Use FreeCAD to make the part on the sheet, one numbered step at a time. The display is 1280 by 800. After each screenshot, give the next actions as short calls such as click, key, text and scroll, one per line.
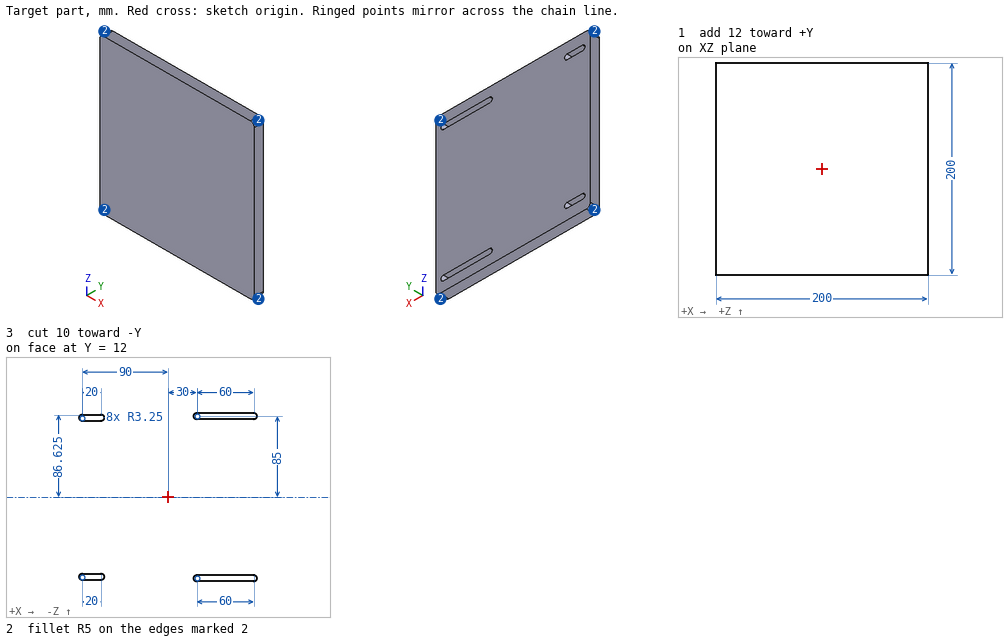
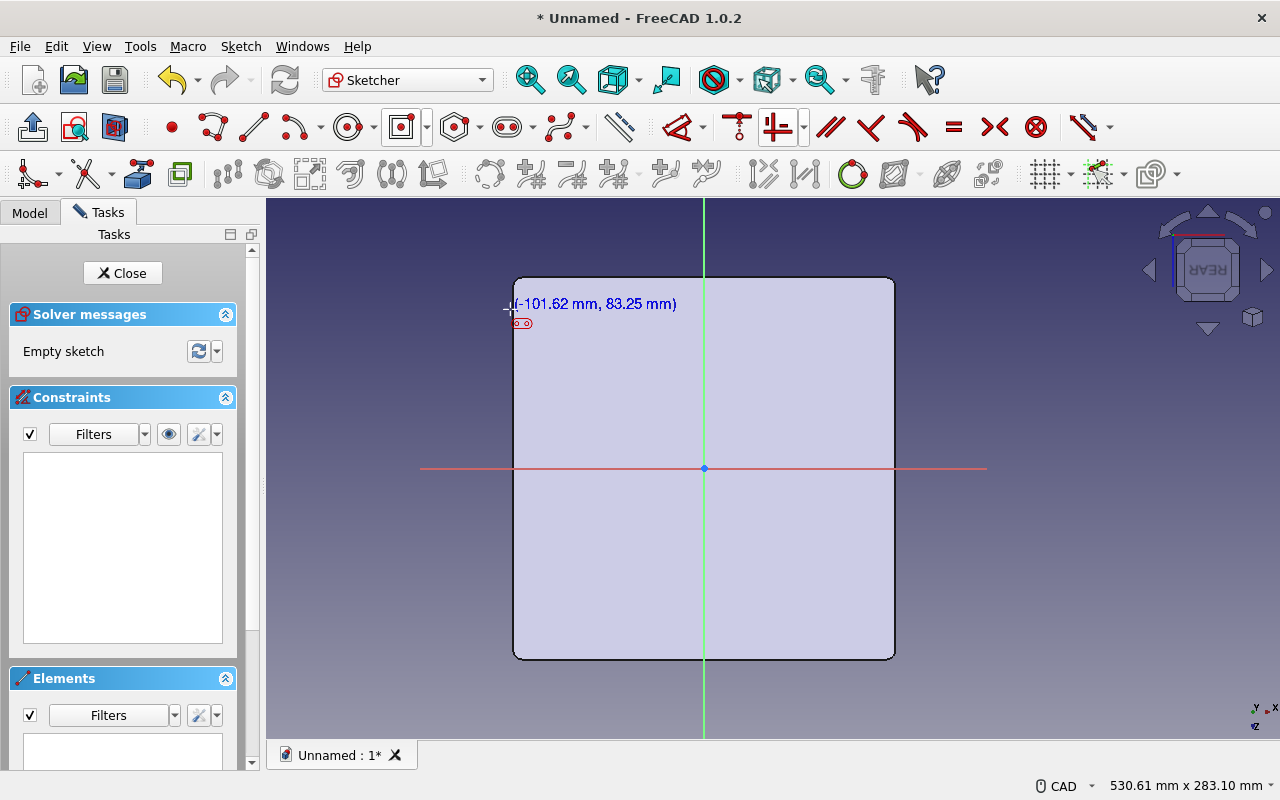
click(532, 309)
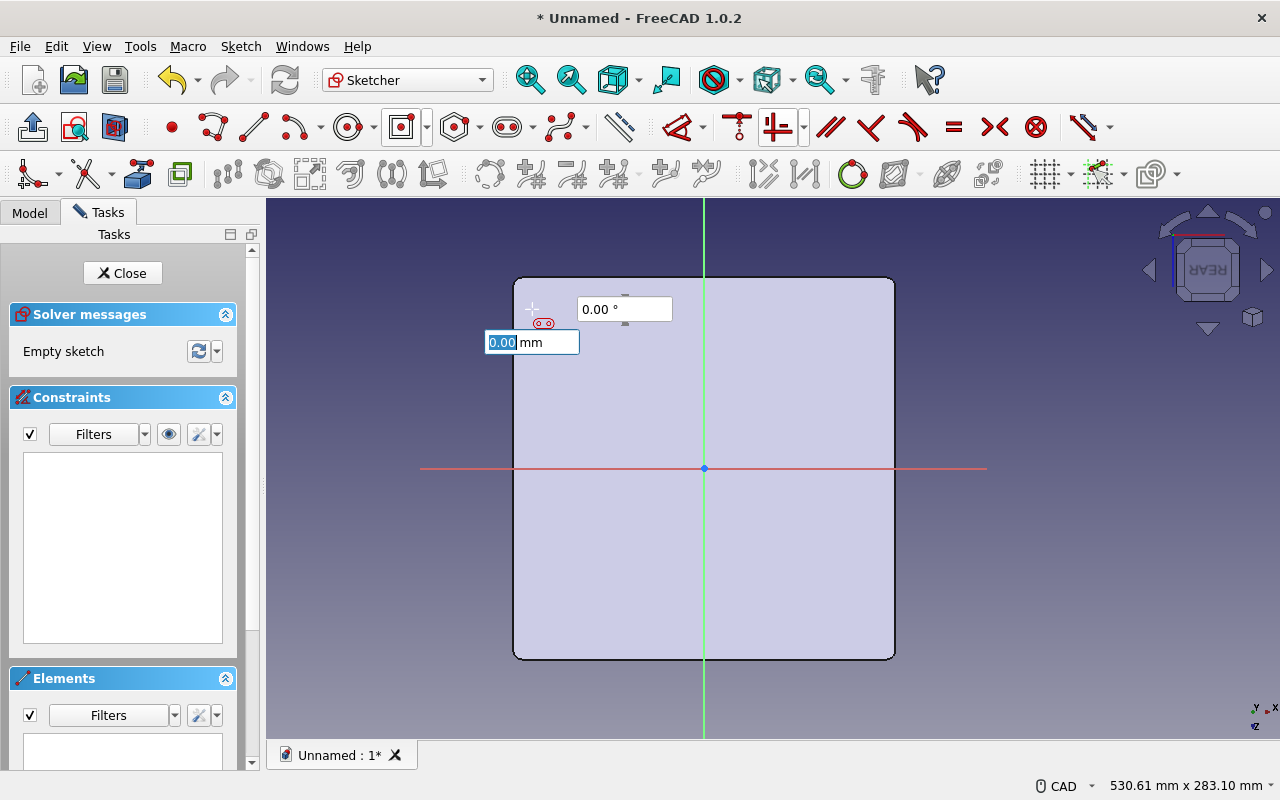
click(571, 309)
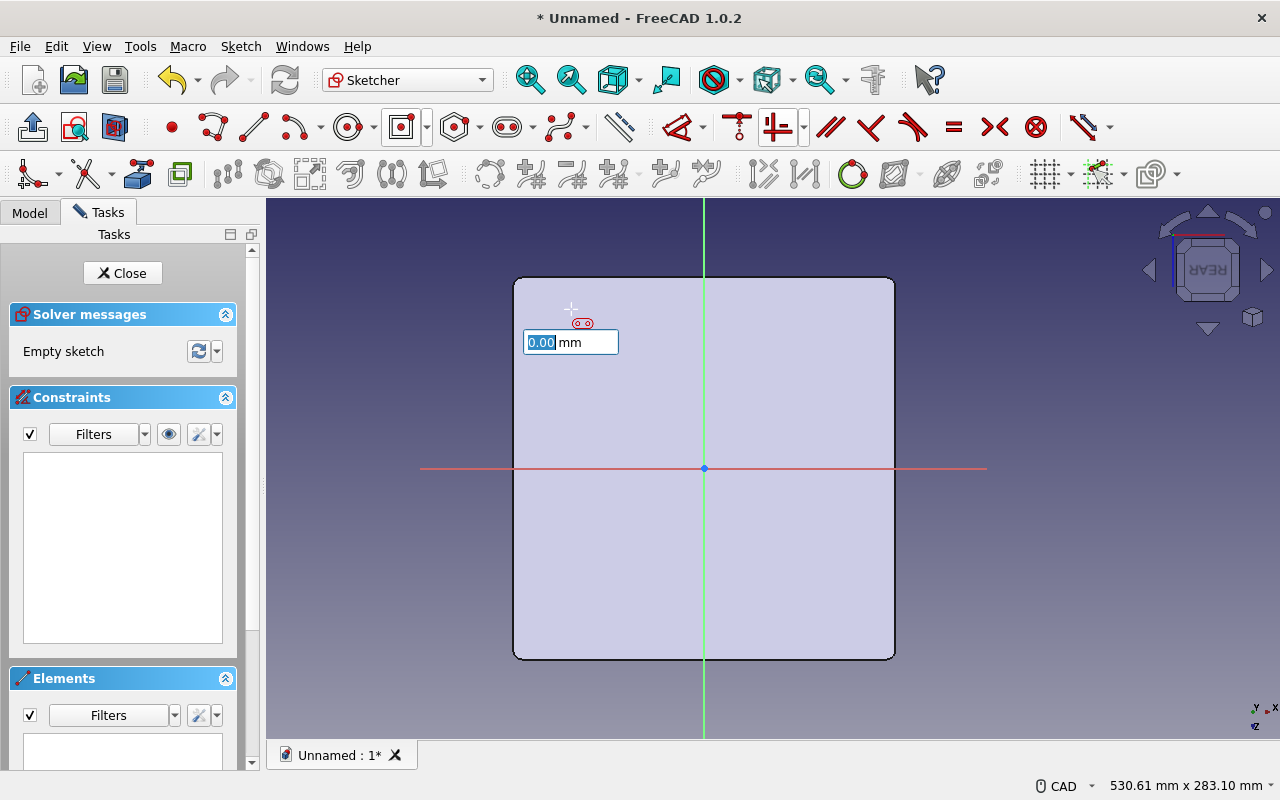
scroll(551, 303, up, 5)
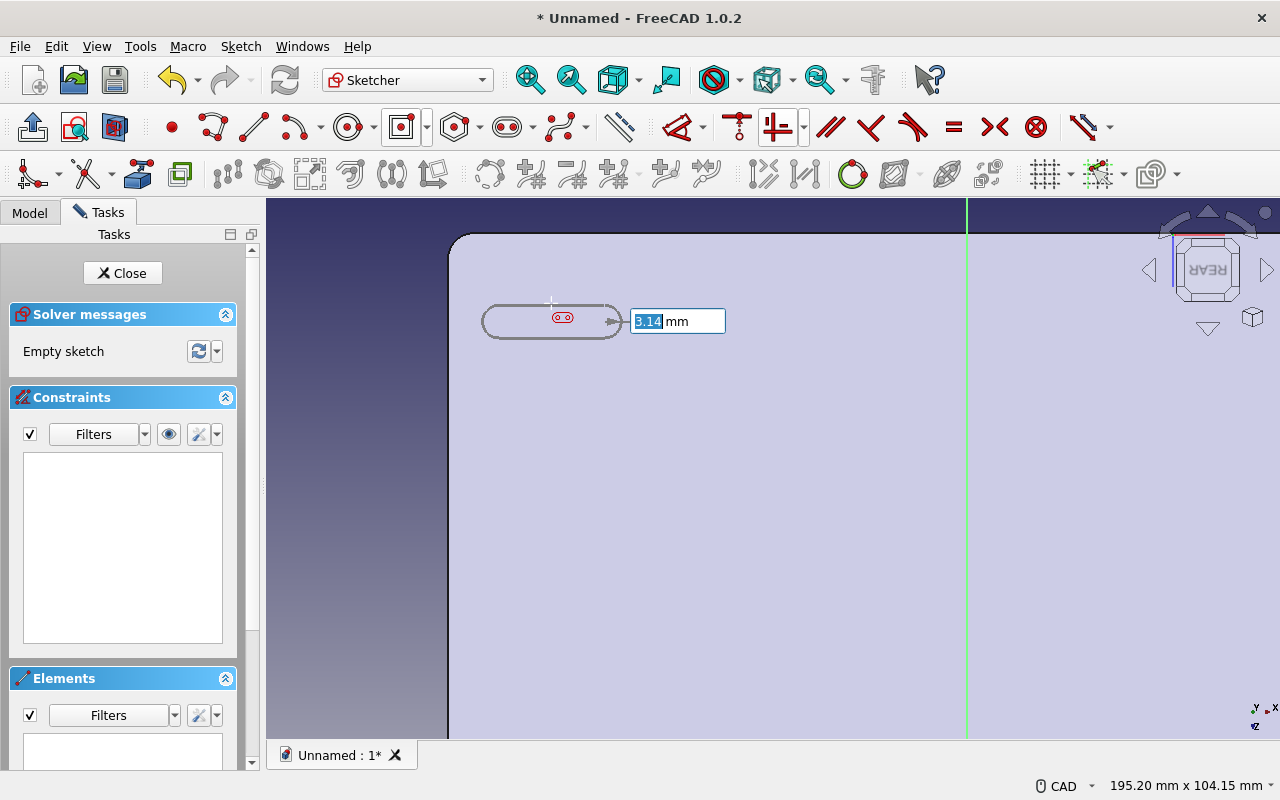
click(552, 303)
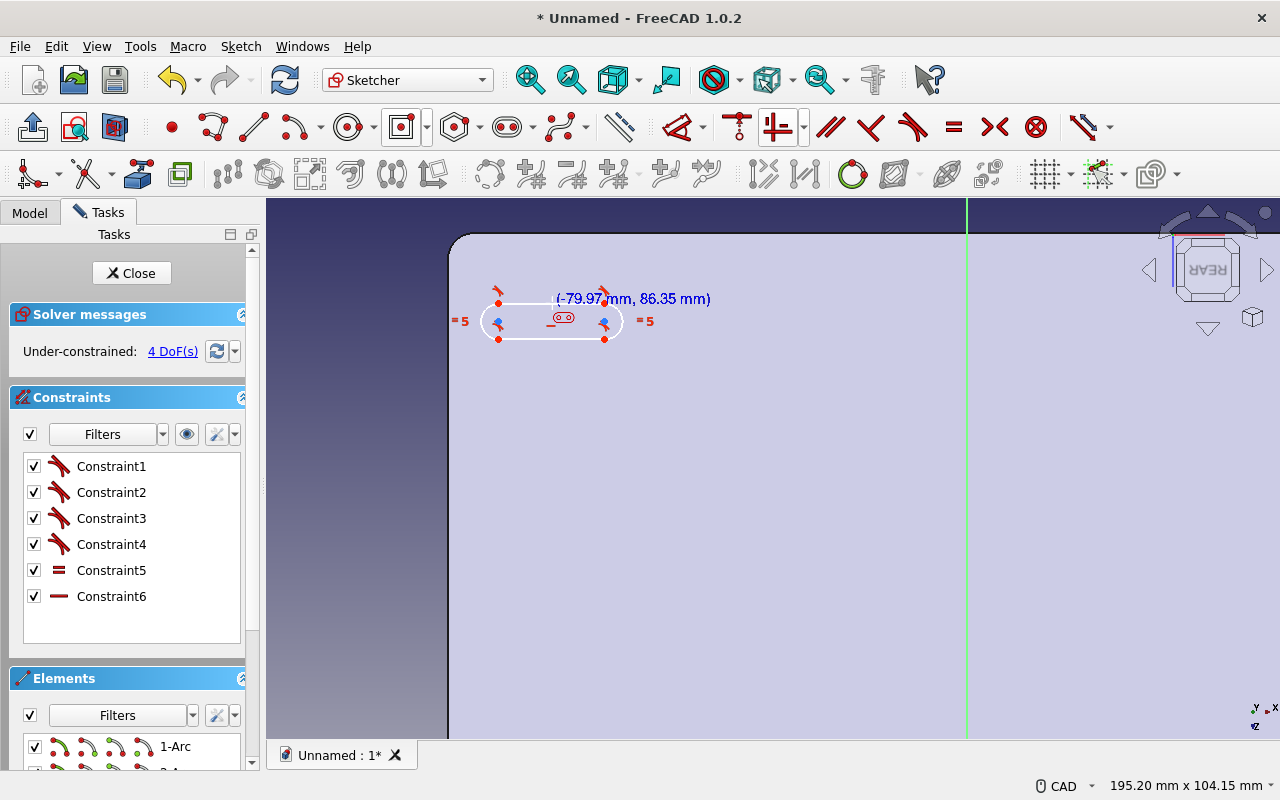
scroll(551, 303, down, 5)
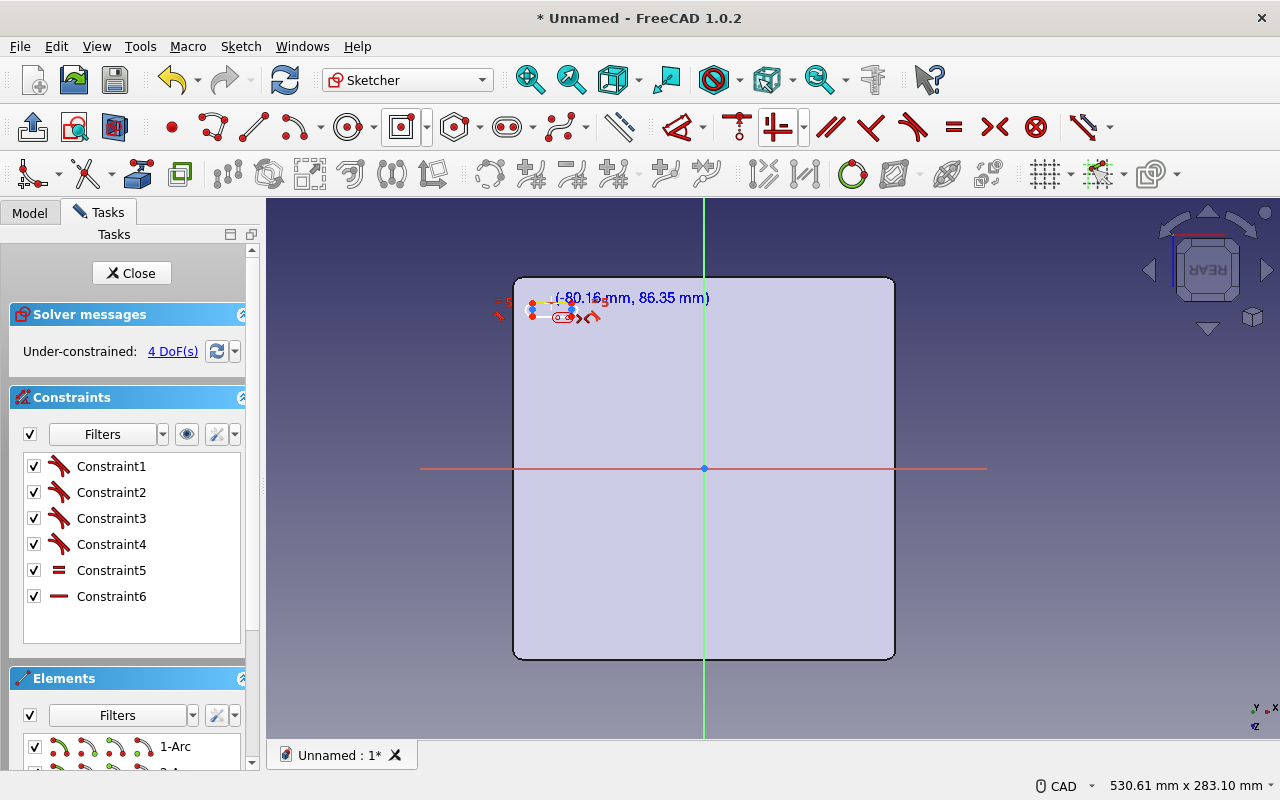
scroll(532, 628, up, 7)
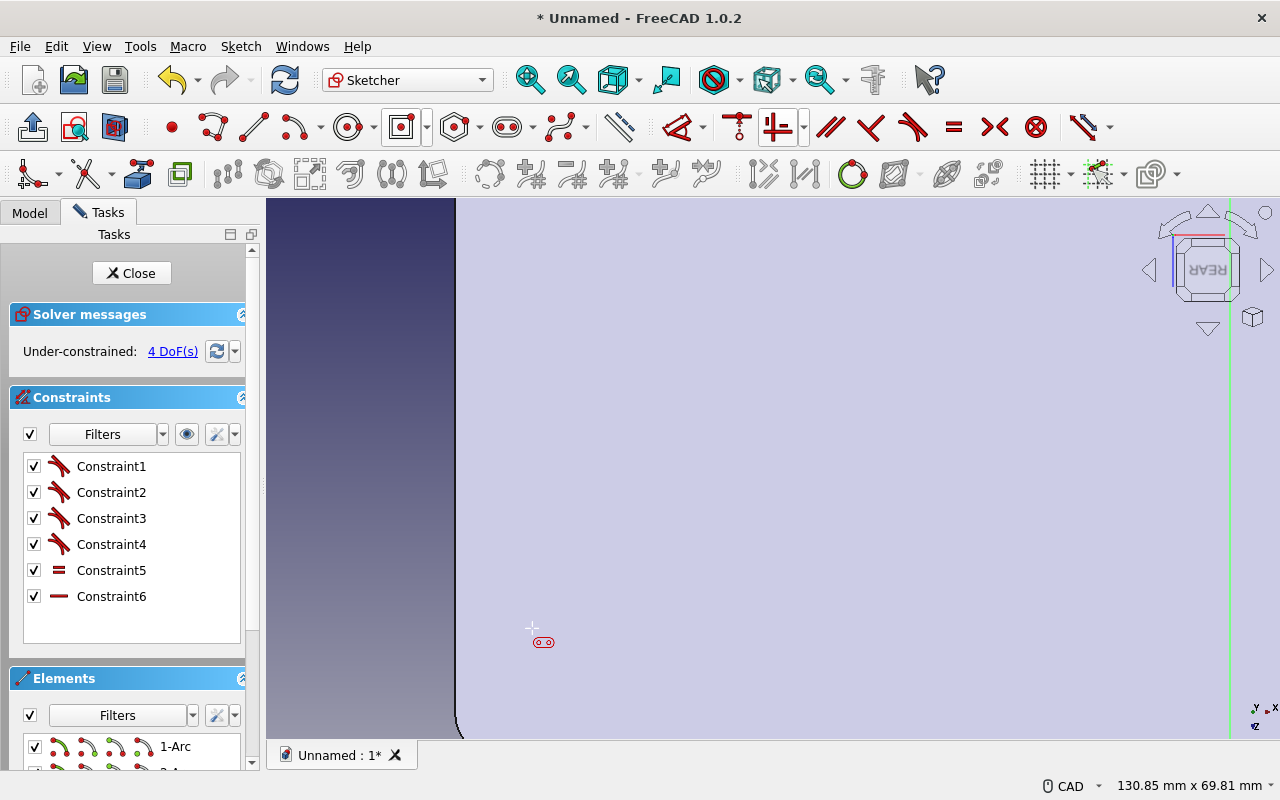
scroll(532, 629, down, 7)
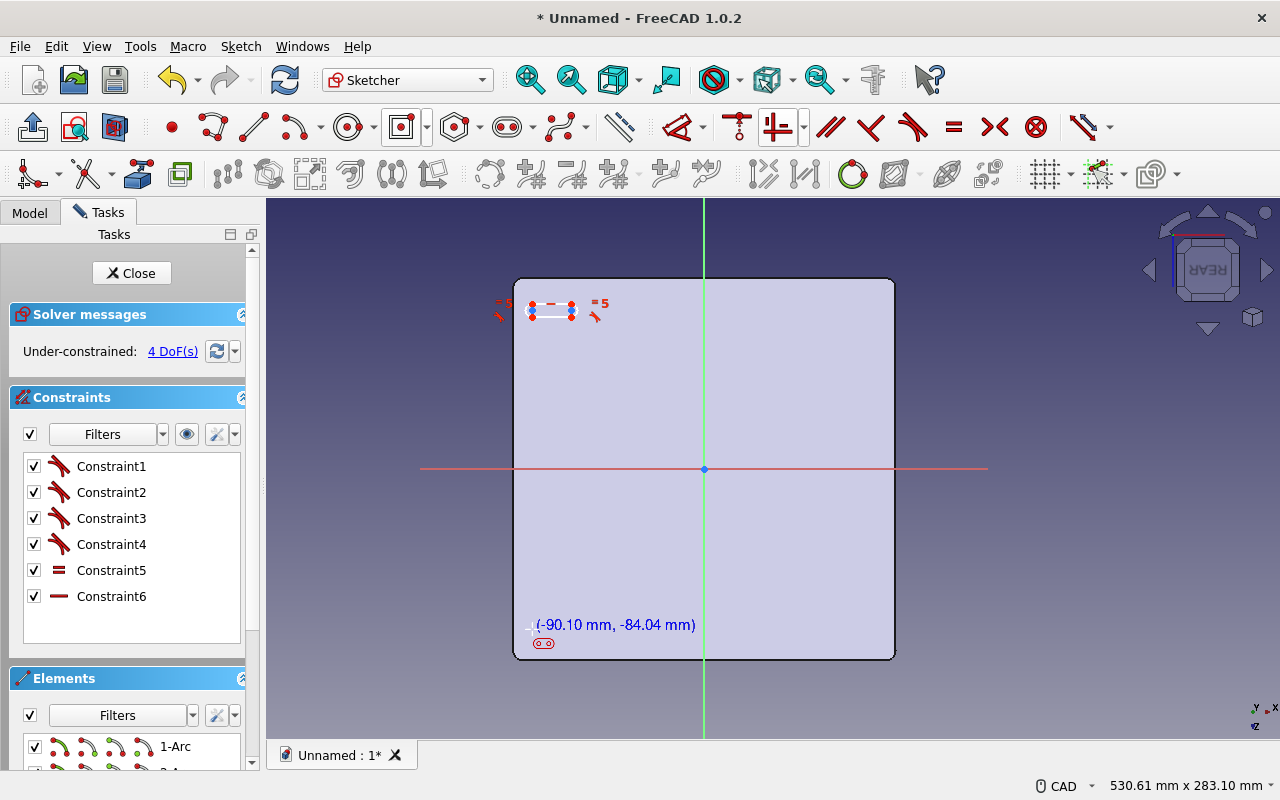
click(532, 629)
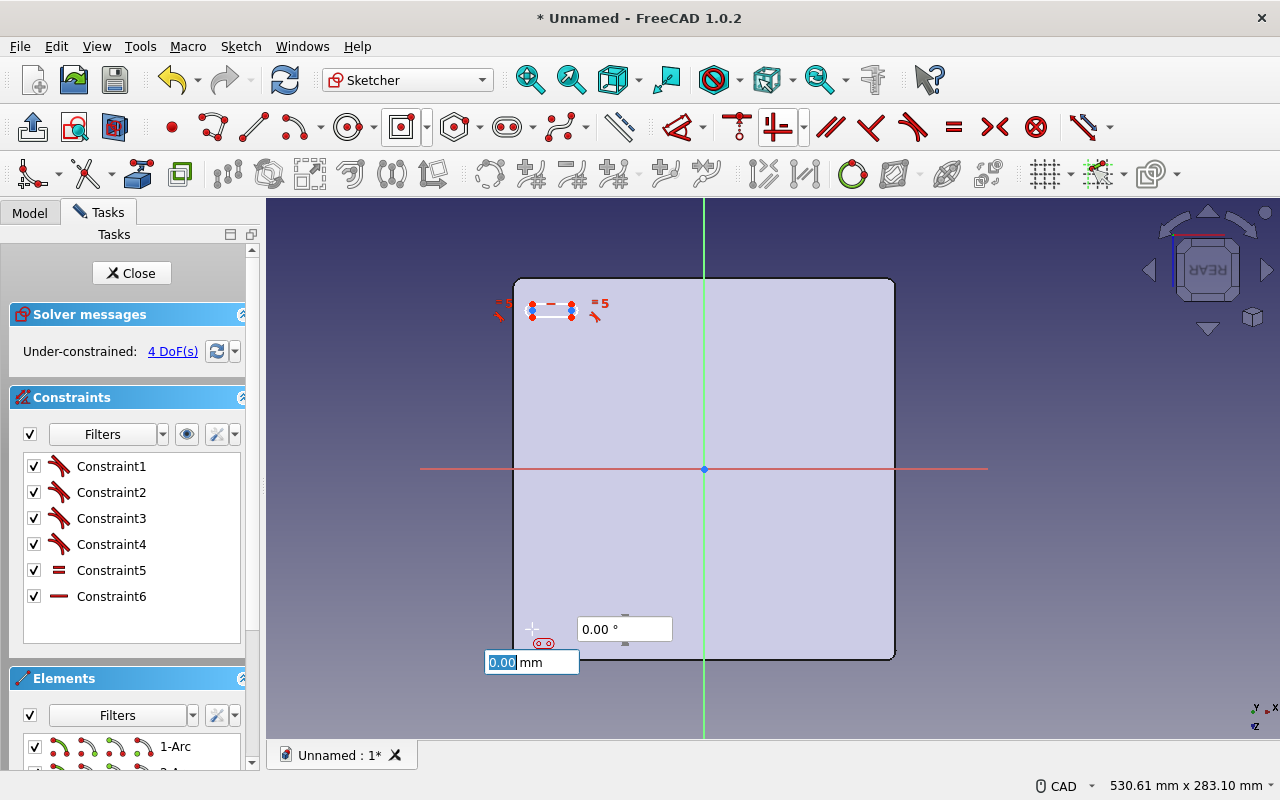
click(571, 629)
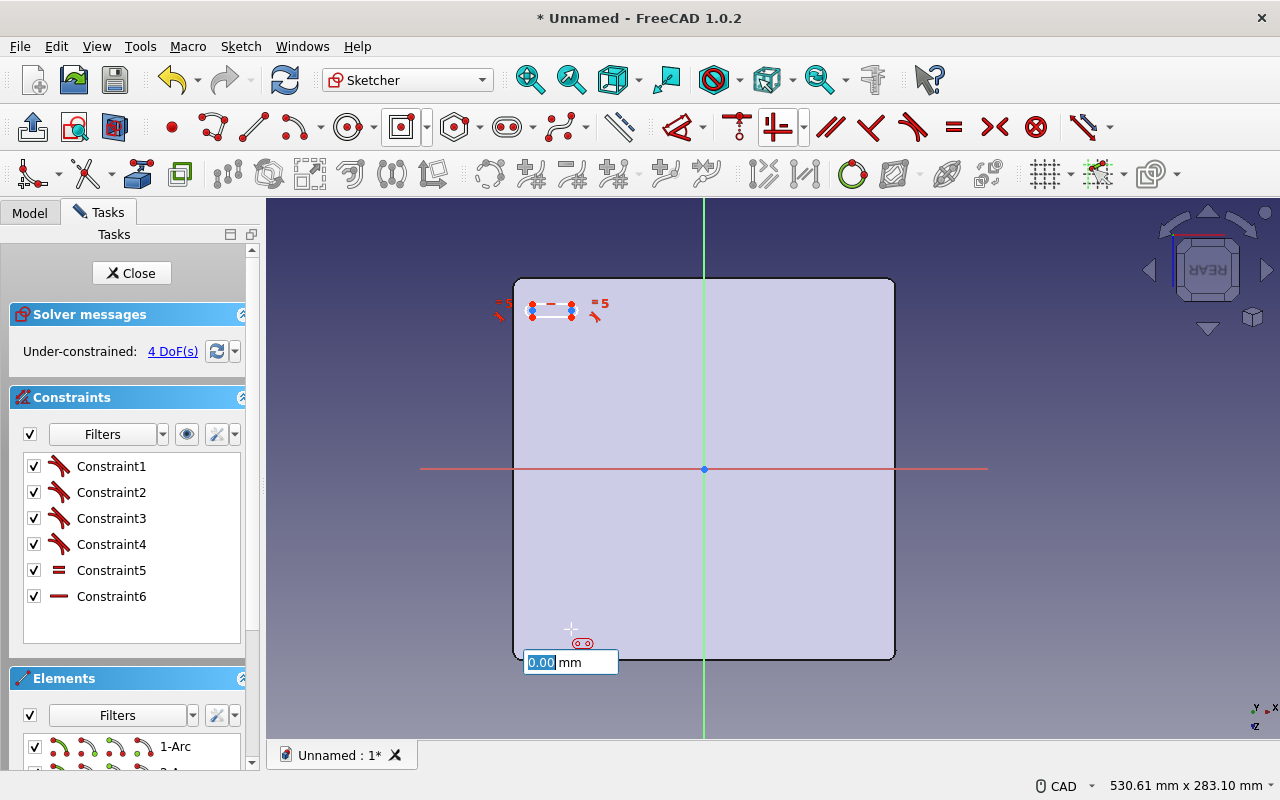
scroll(551, 635, up, 5)